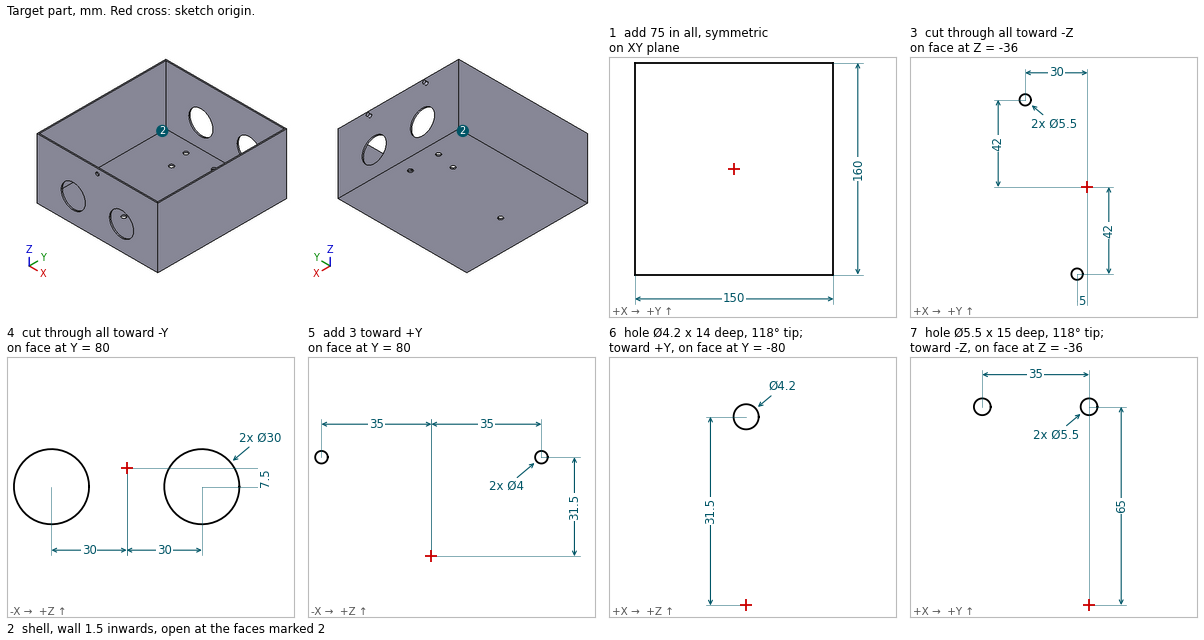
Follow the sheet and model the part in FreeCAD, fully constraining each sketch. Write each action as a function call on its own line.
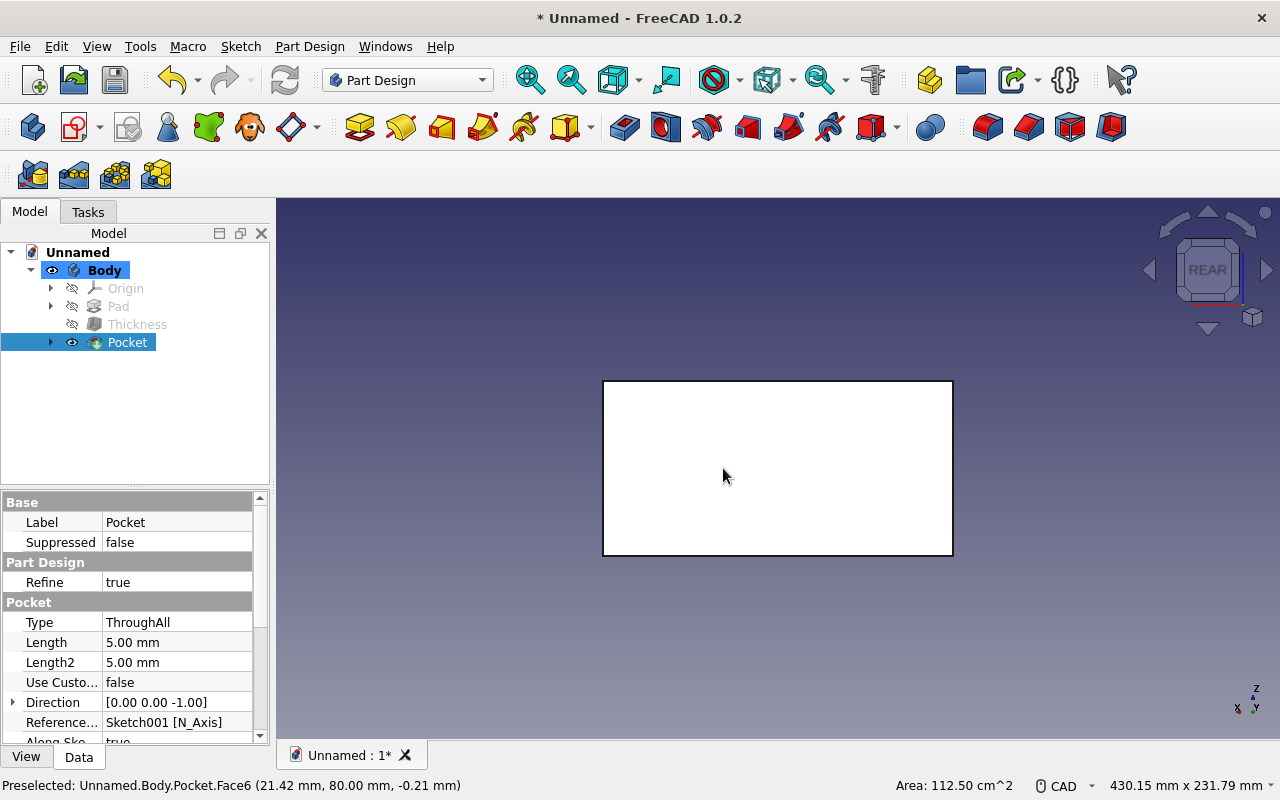
click(74, 128)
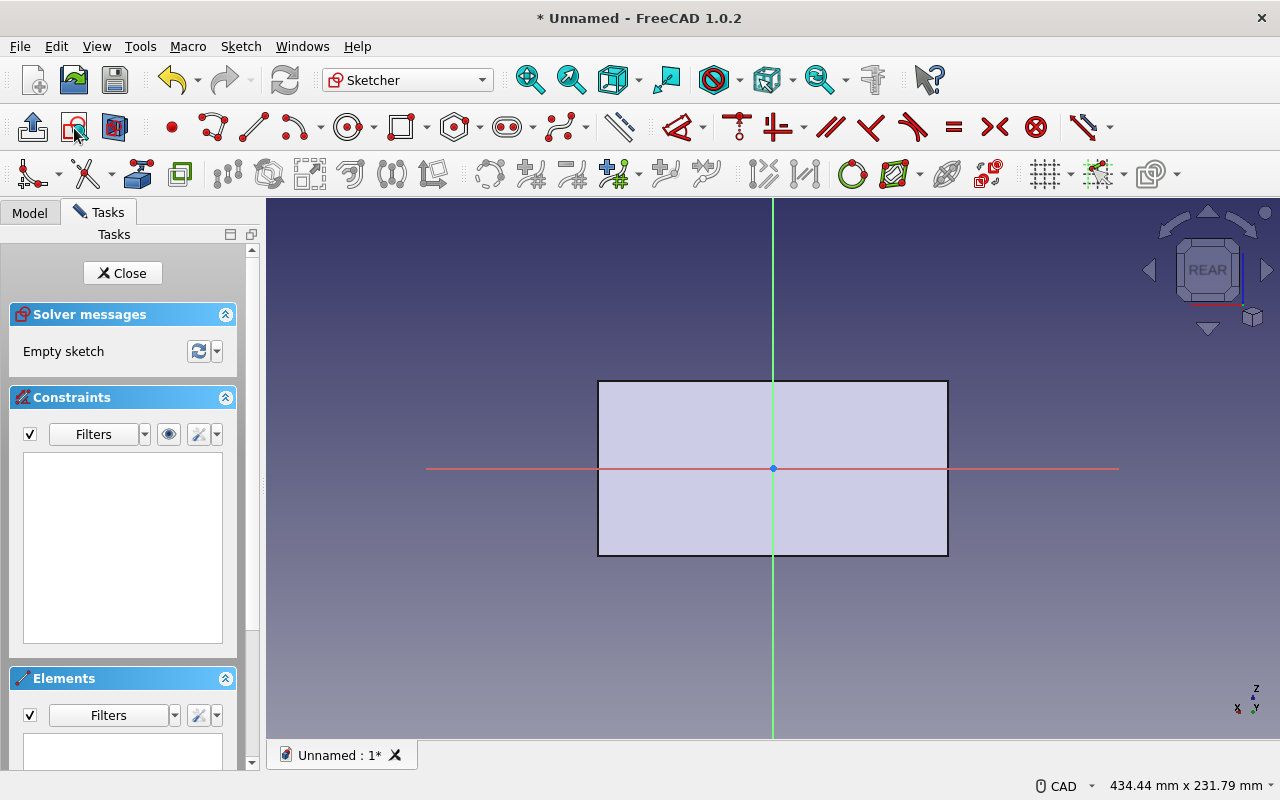
scroll(813, 496, up, 5)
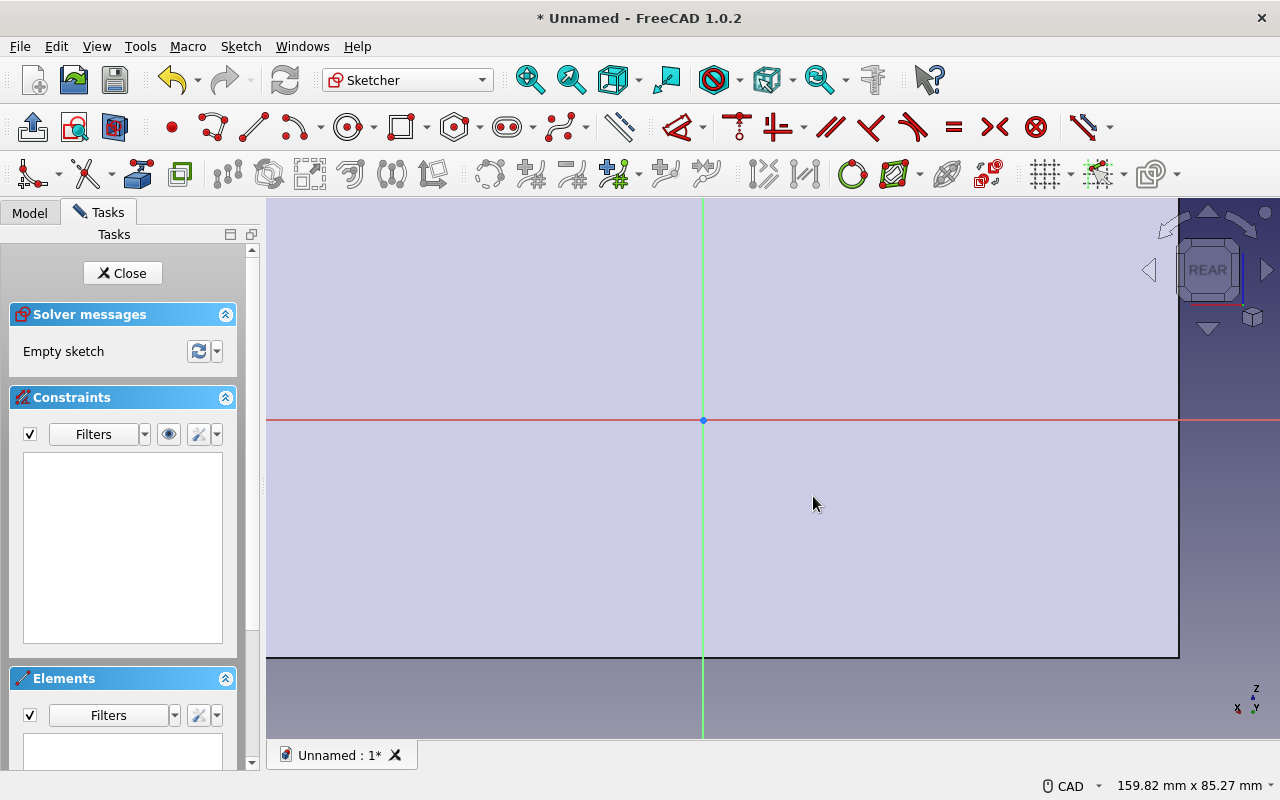
key(g)
key(c)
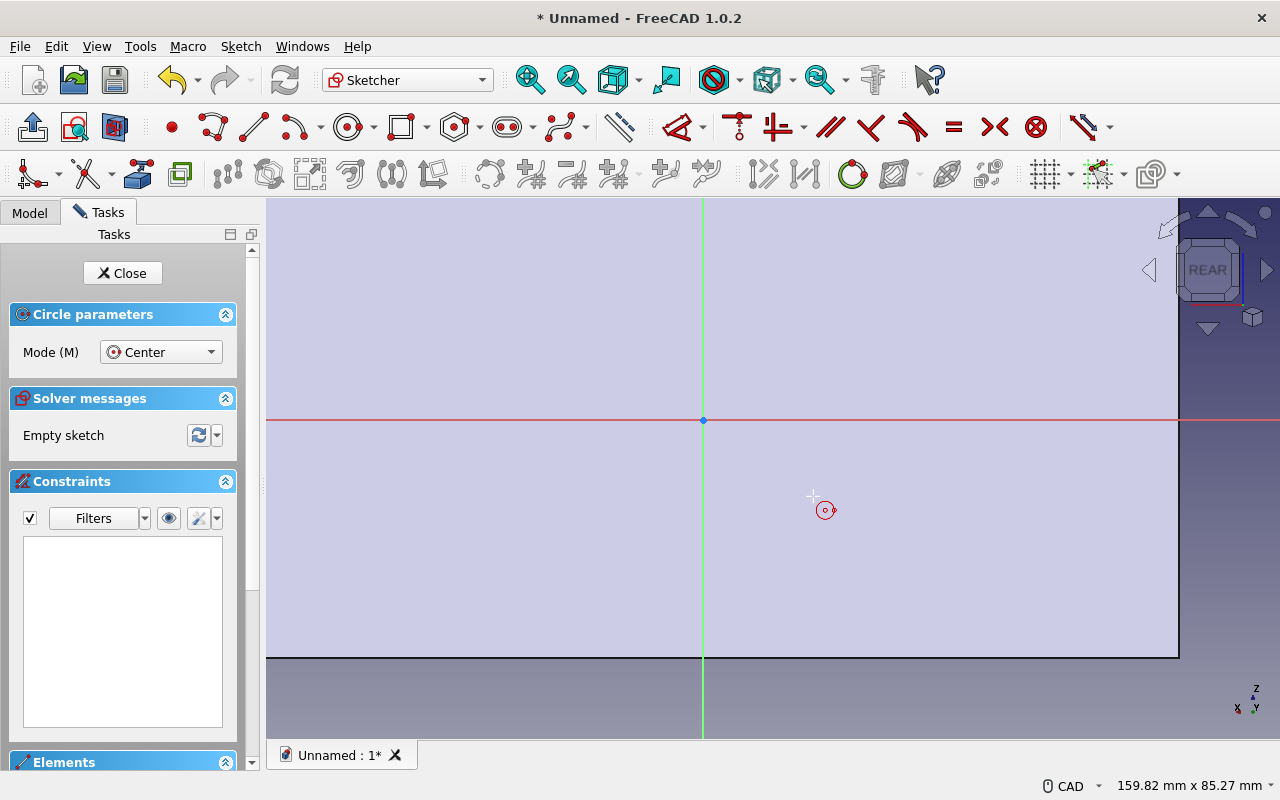
click(894, 468)
move(961, 401)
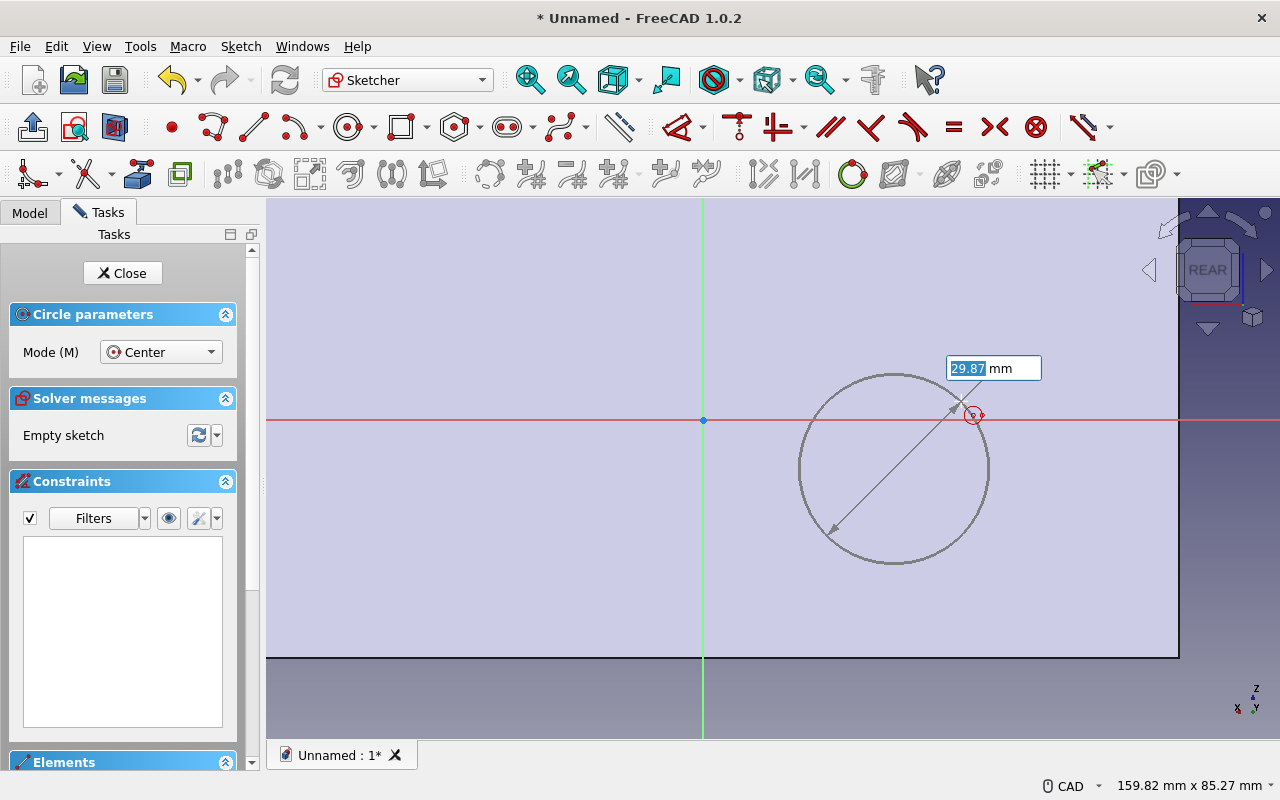
text(30)
key(Return)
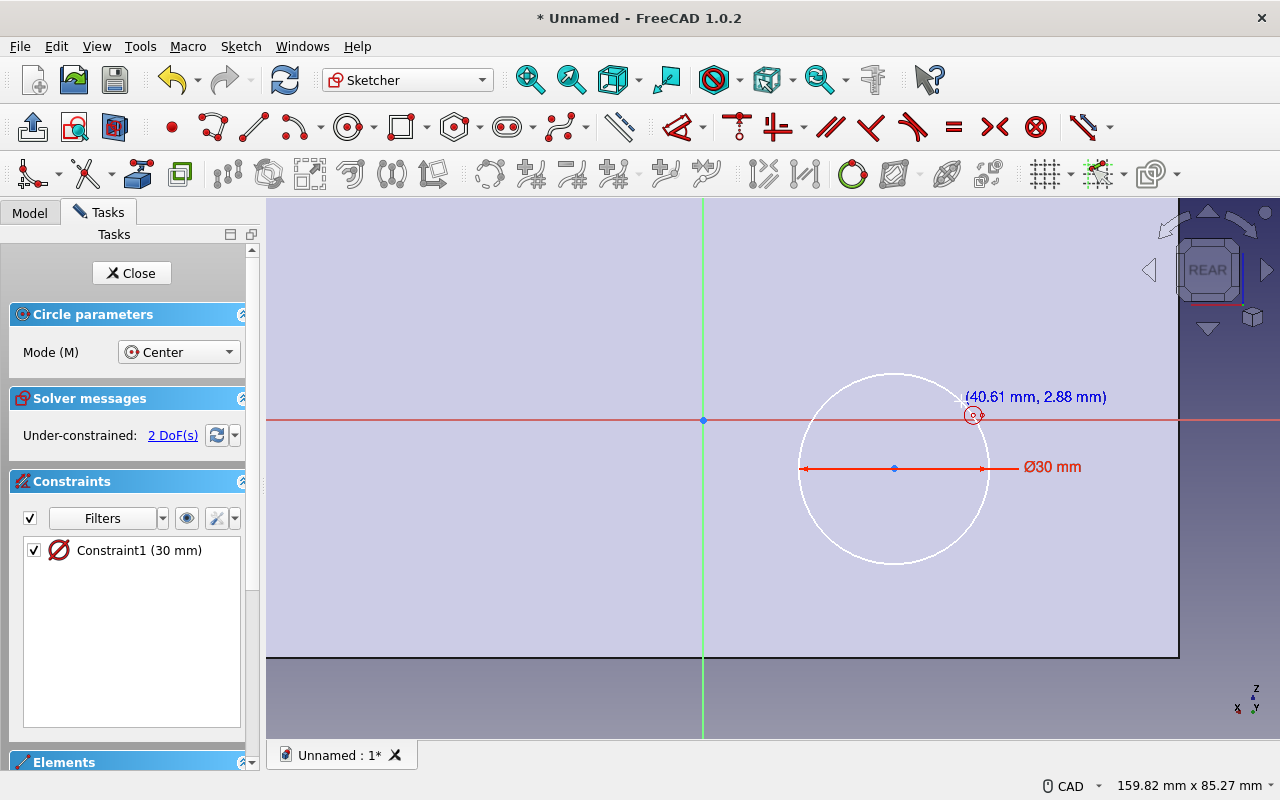
click(513, 468)
move(580, 401)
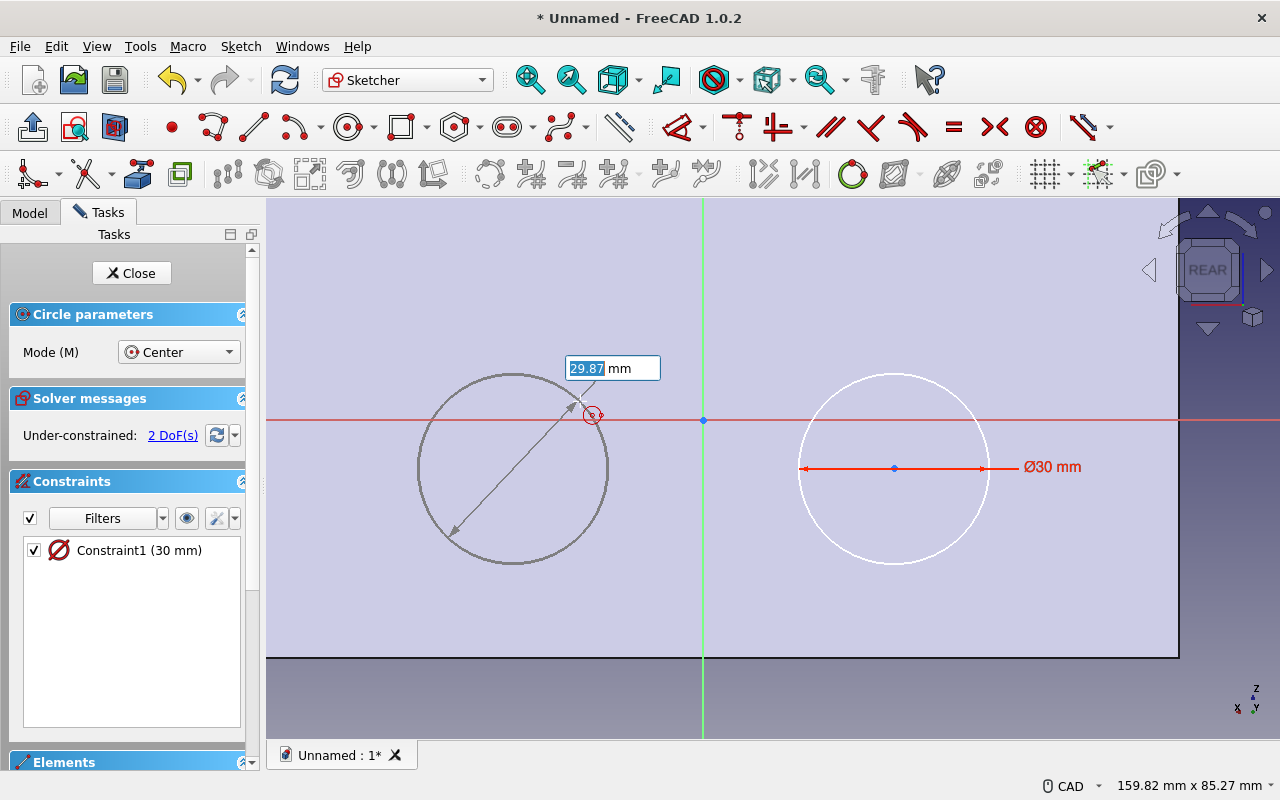
text(30)
key(Return)
key(Escape)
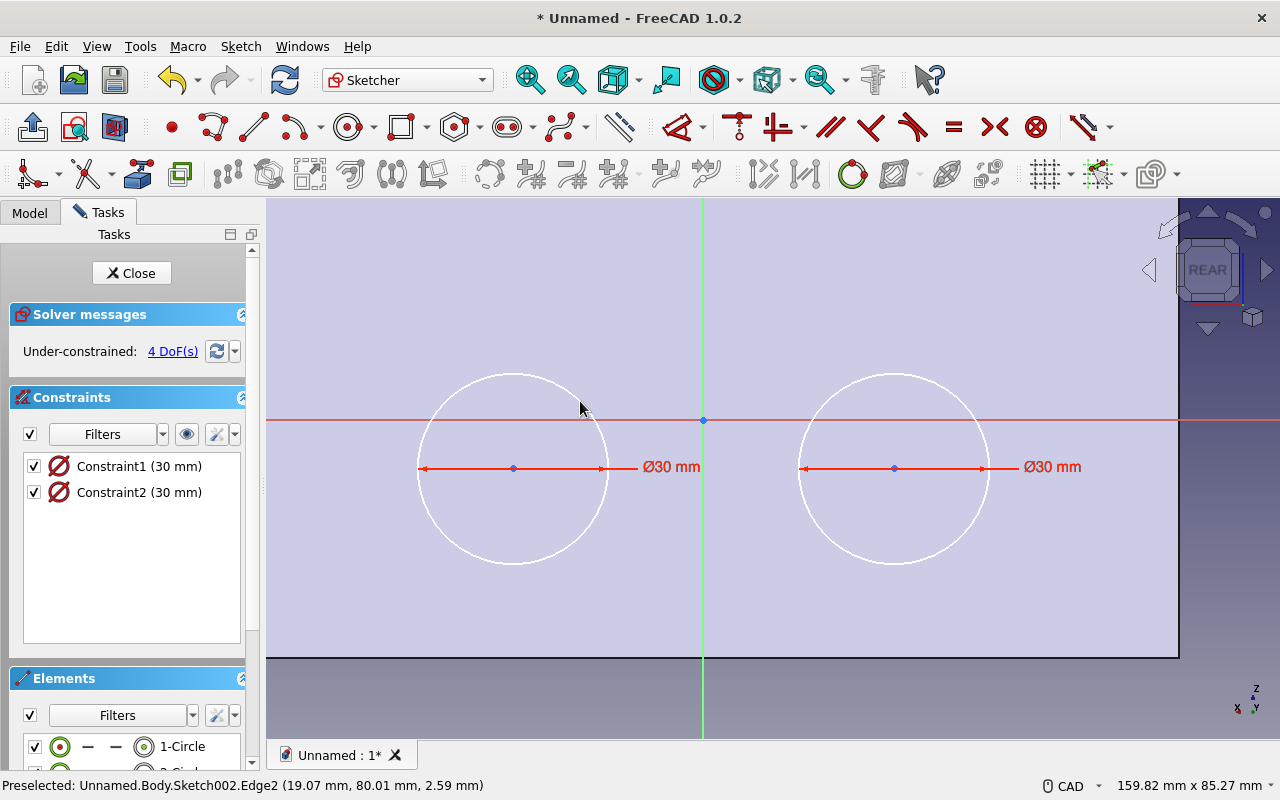
click(894, 469)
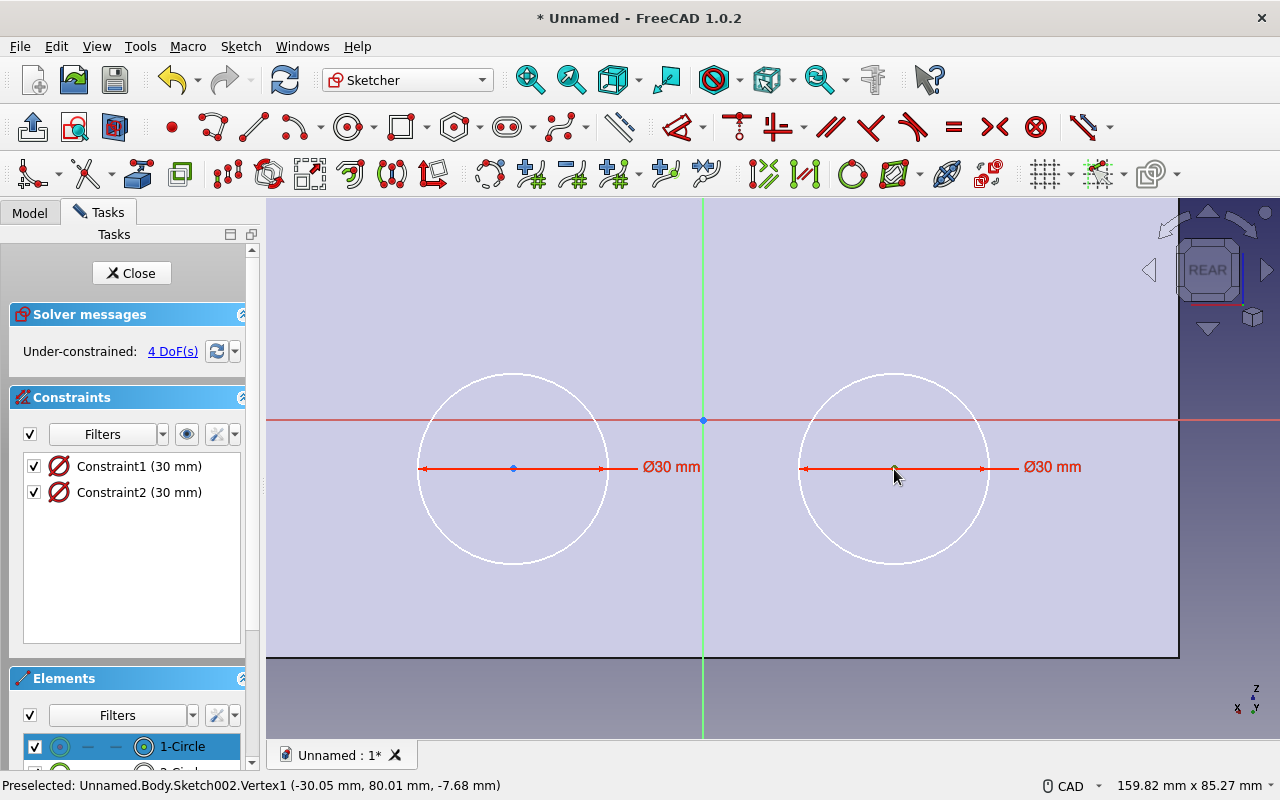
click(513, 469)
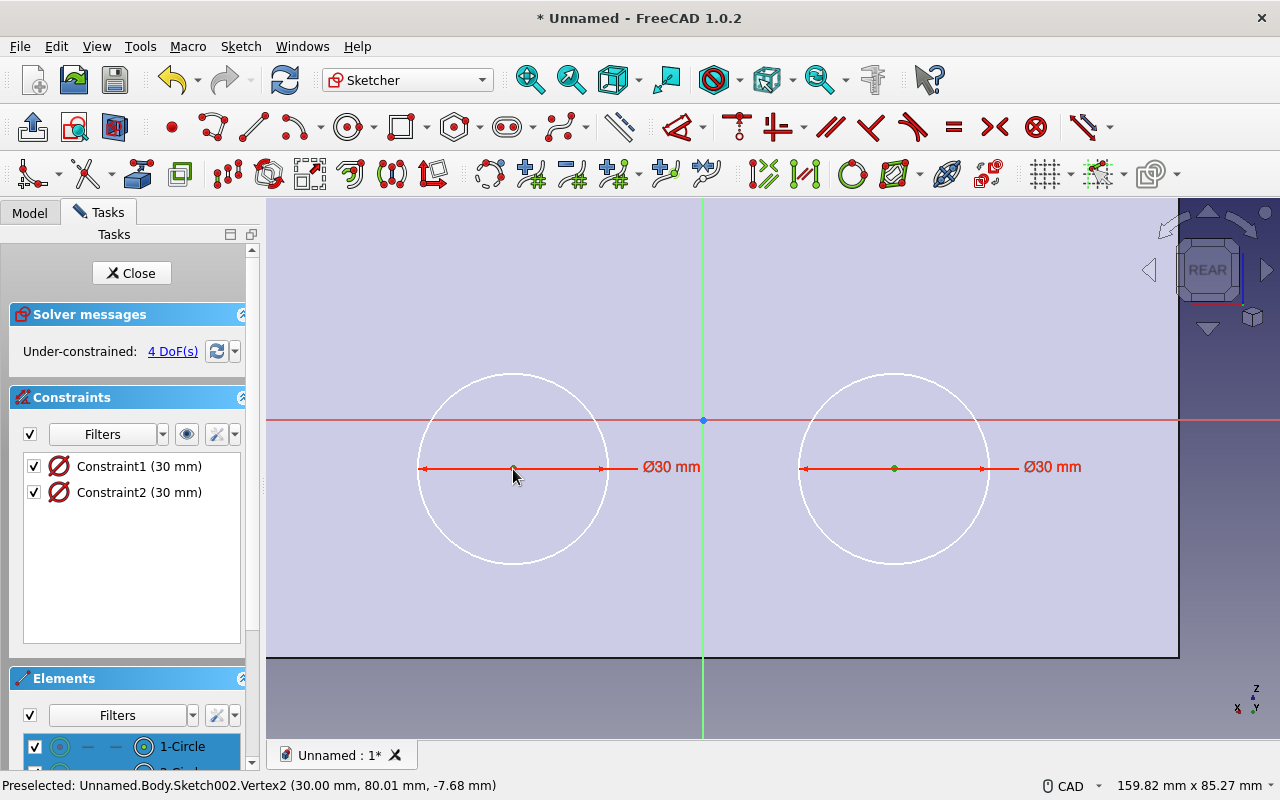
key(h)